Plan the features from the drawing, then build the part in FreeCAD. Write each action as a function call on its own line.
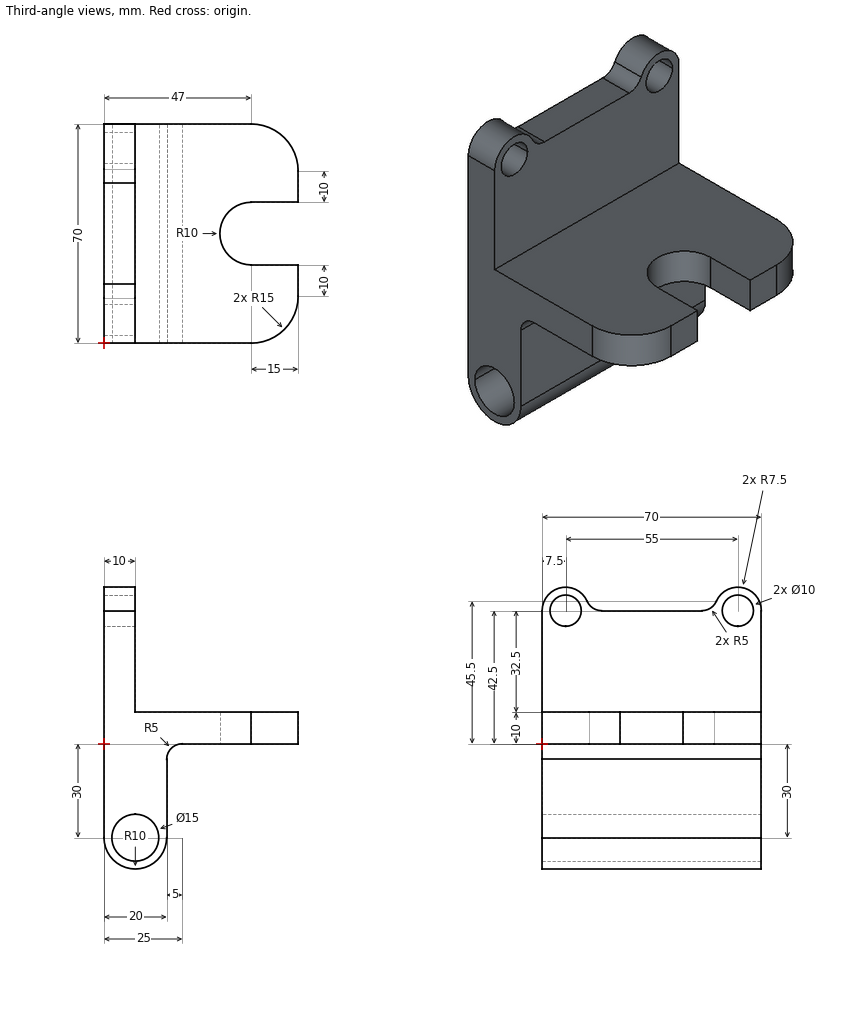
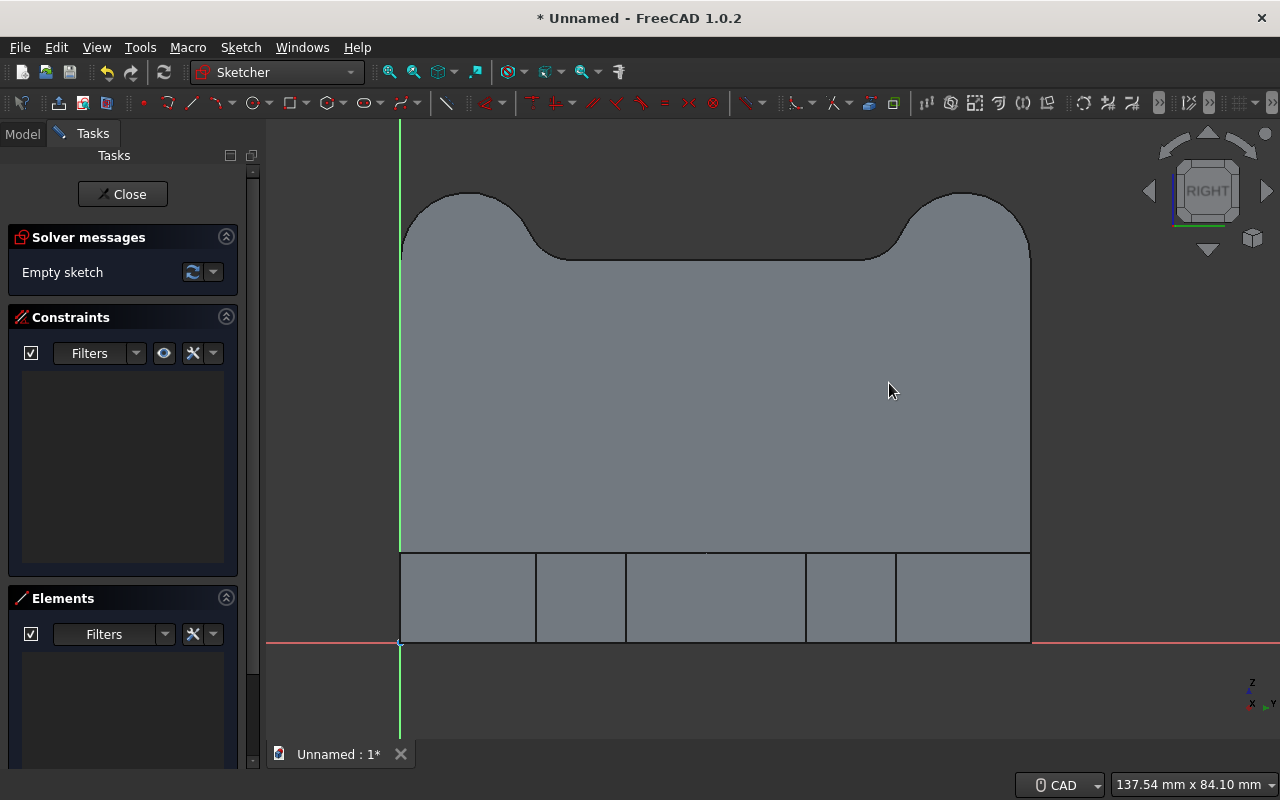
click(254, 104)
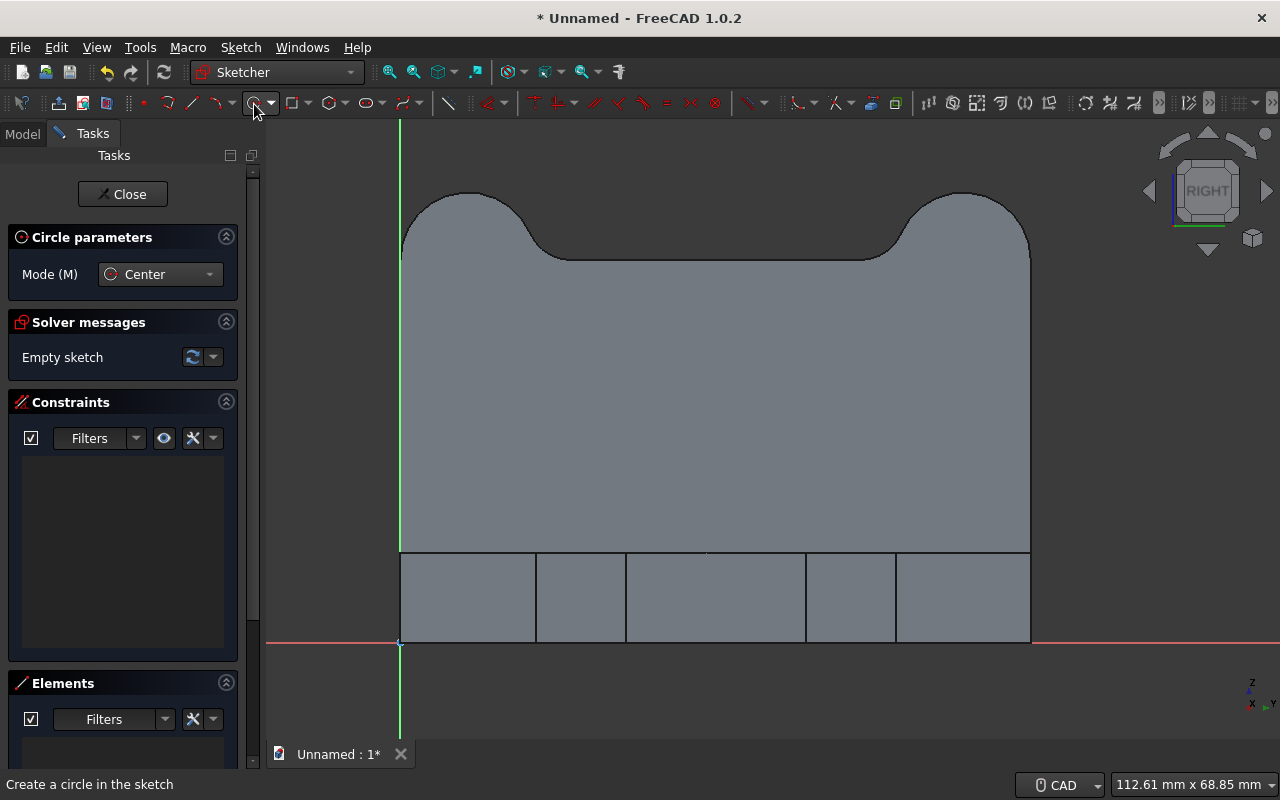
click(963, 260)
click(995, 228)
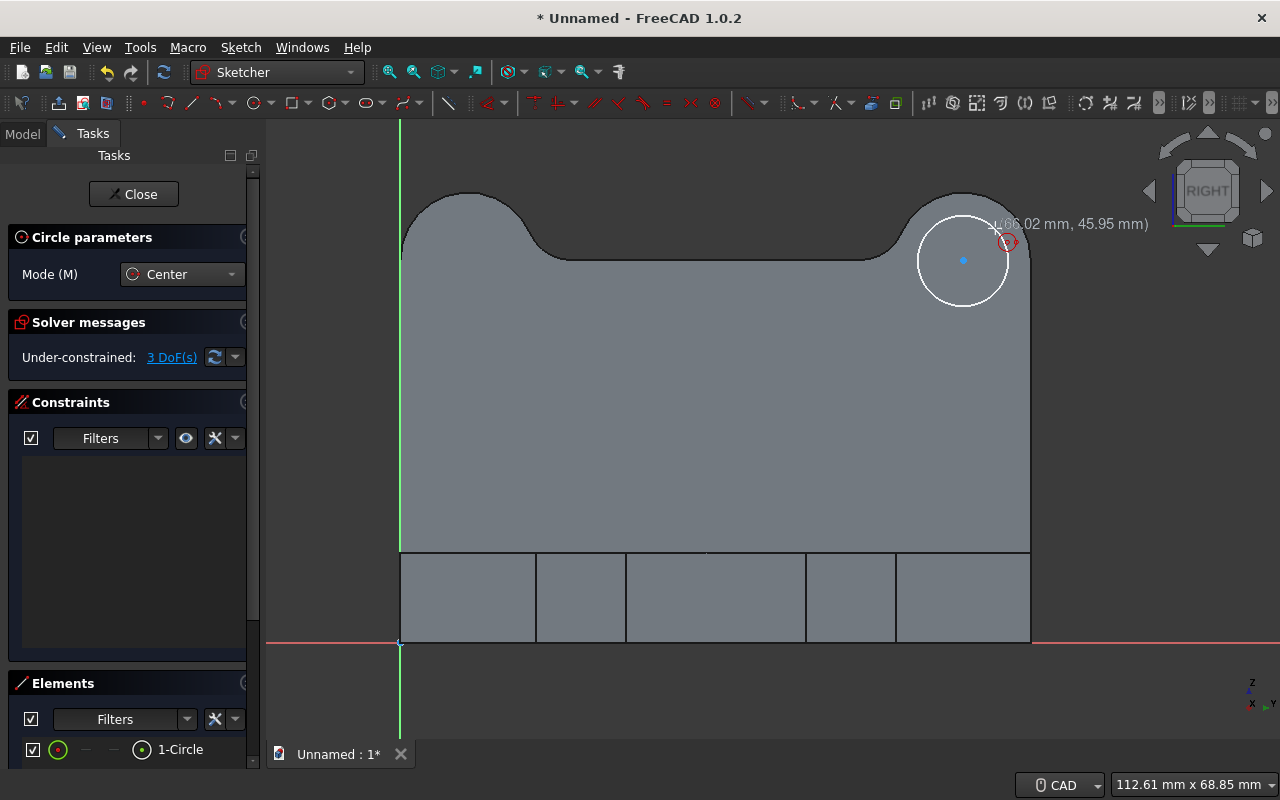
click(468, 260)
click(500, 228)
key(Escape)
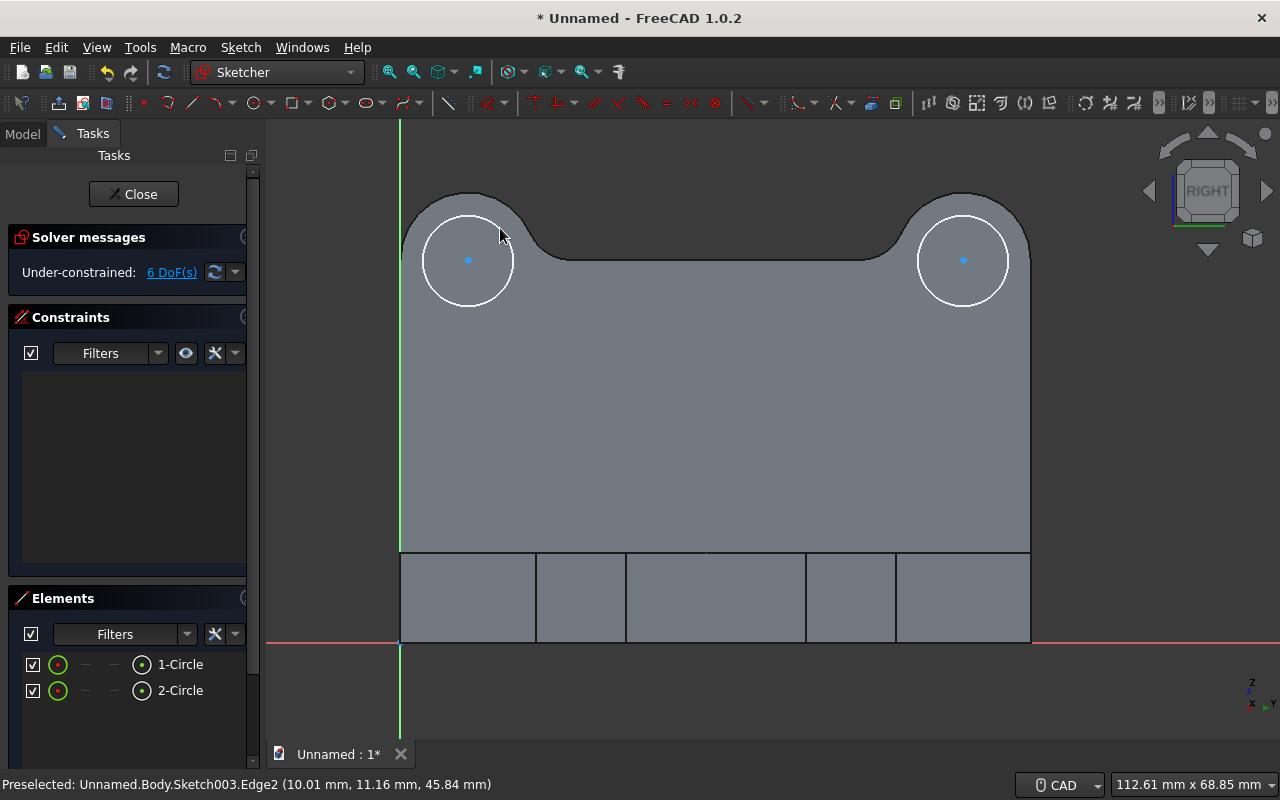
click(995, 229)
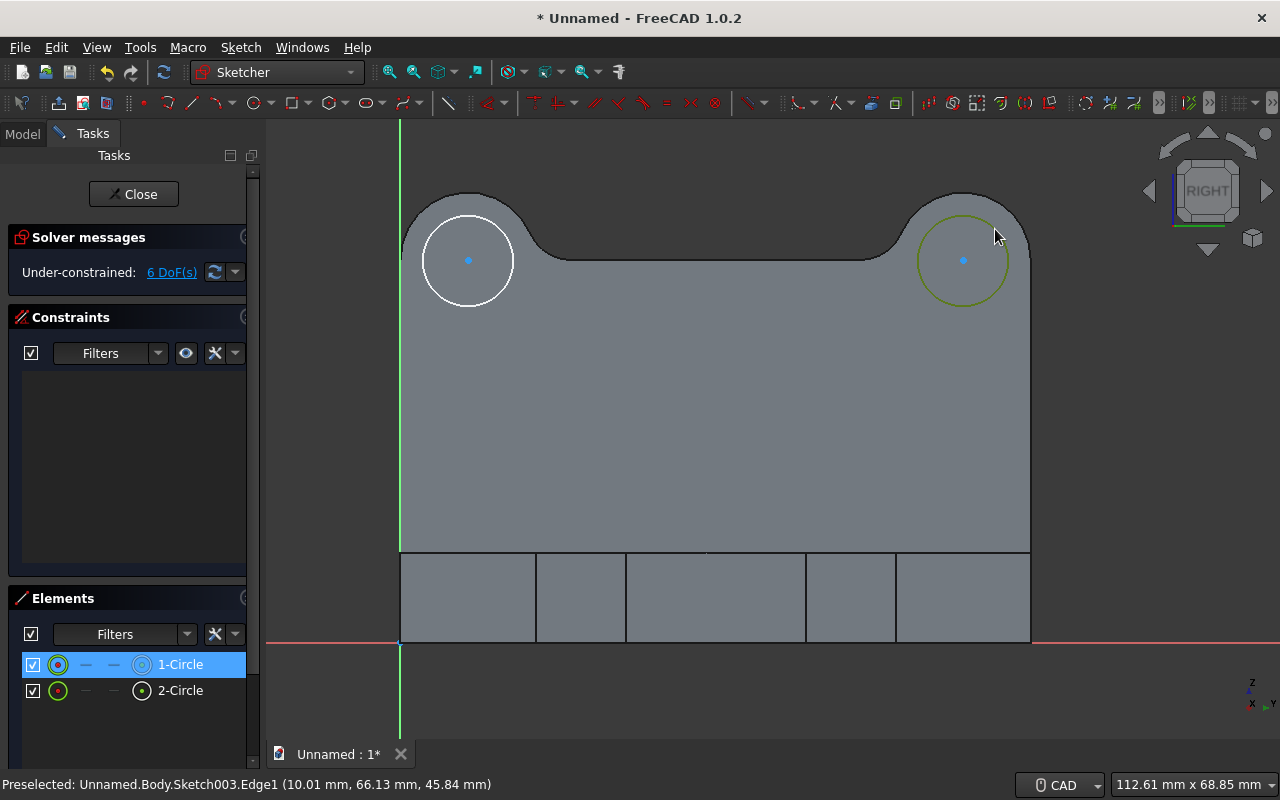
click(500, 229)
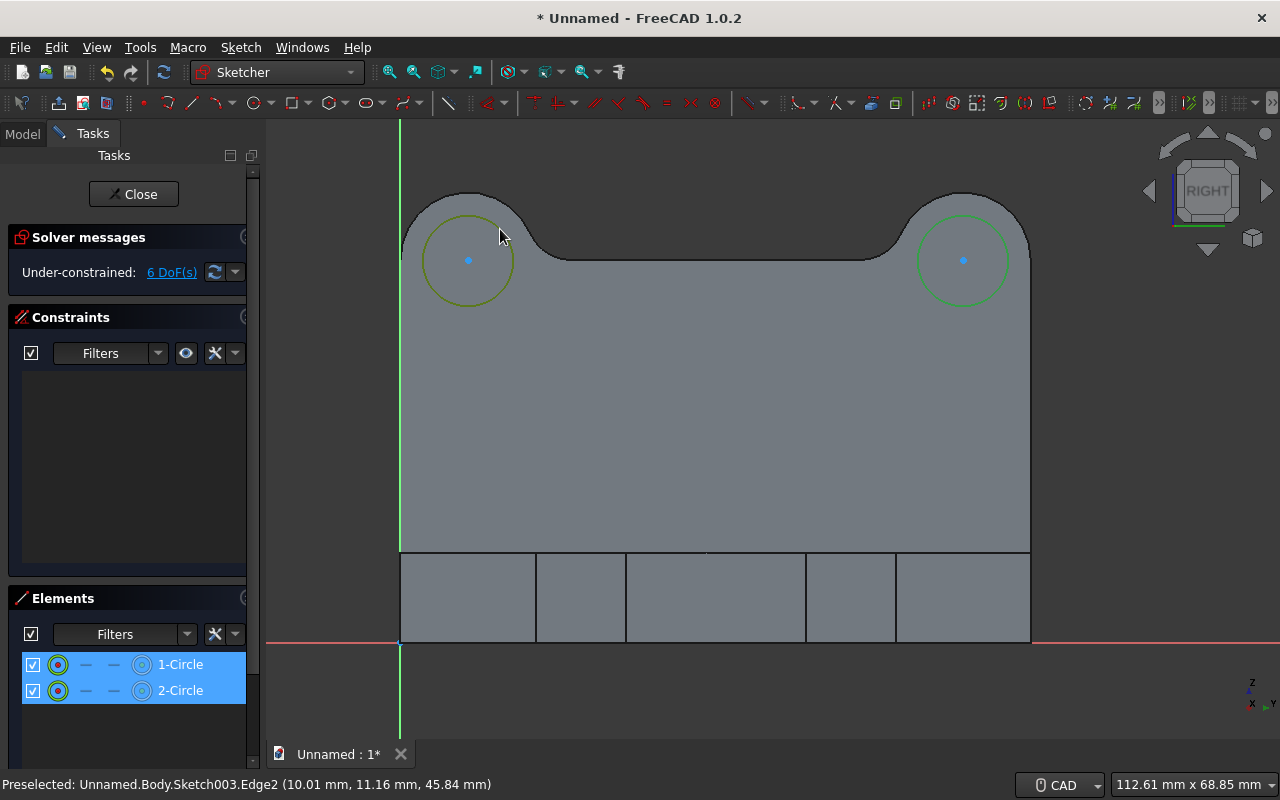
click(668, 104)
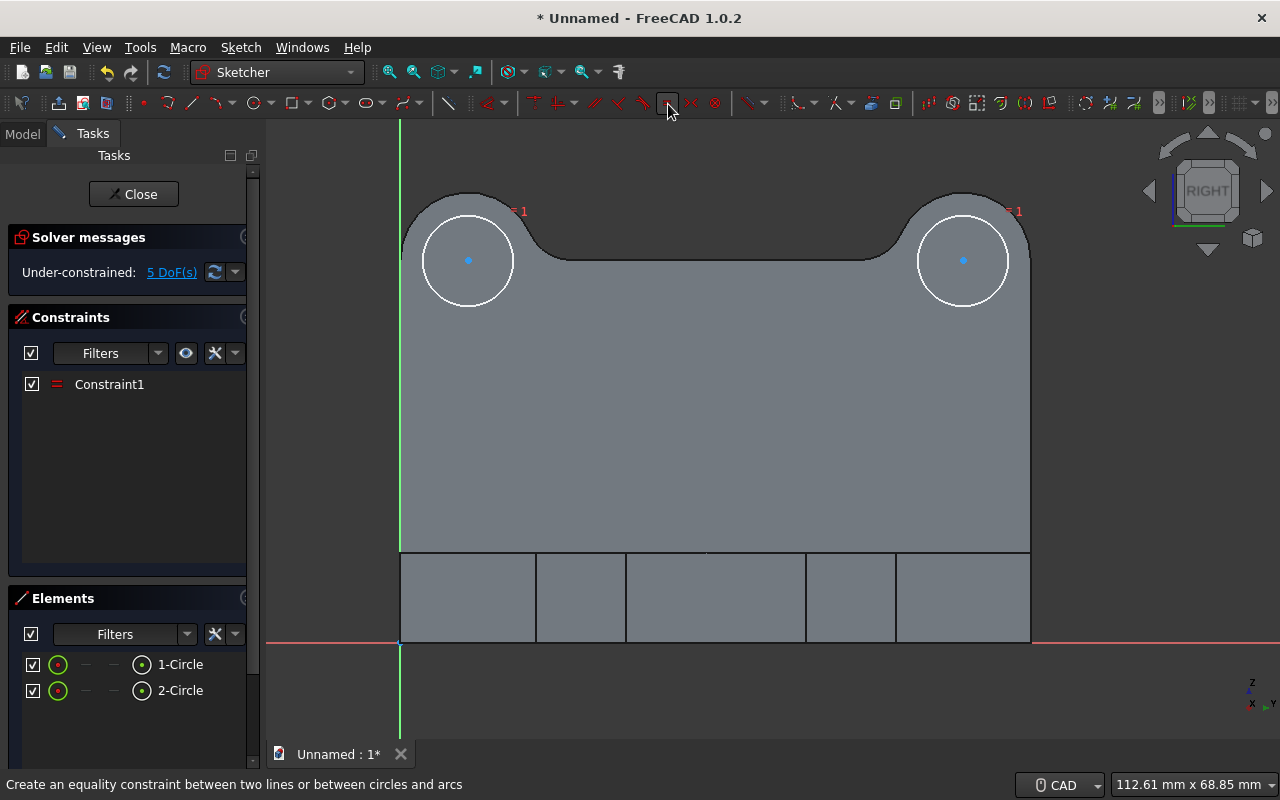
click(963, 261)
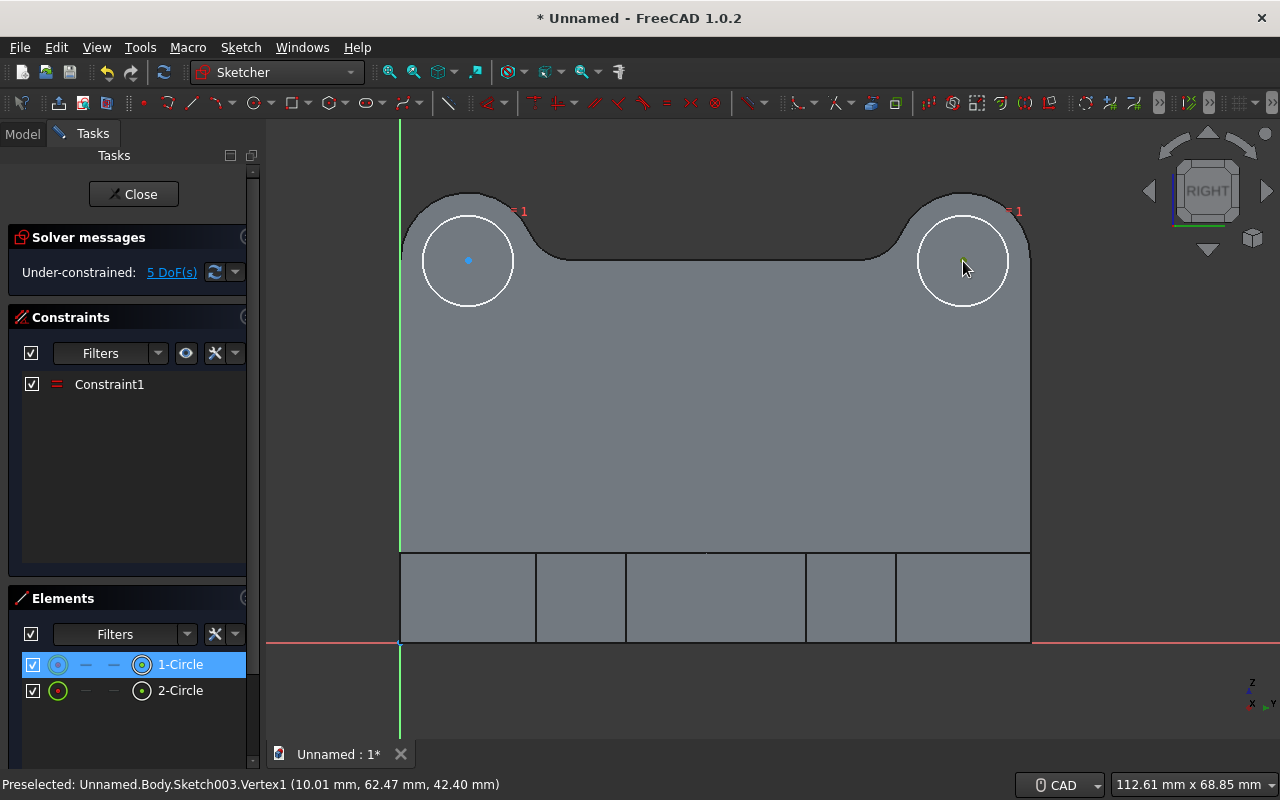
click(468, 261)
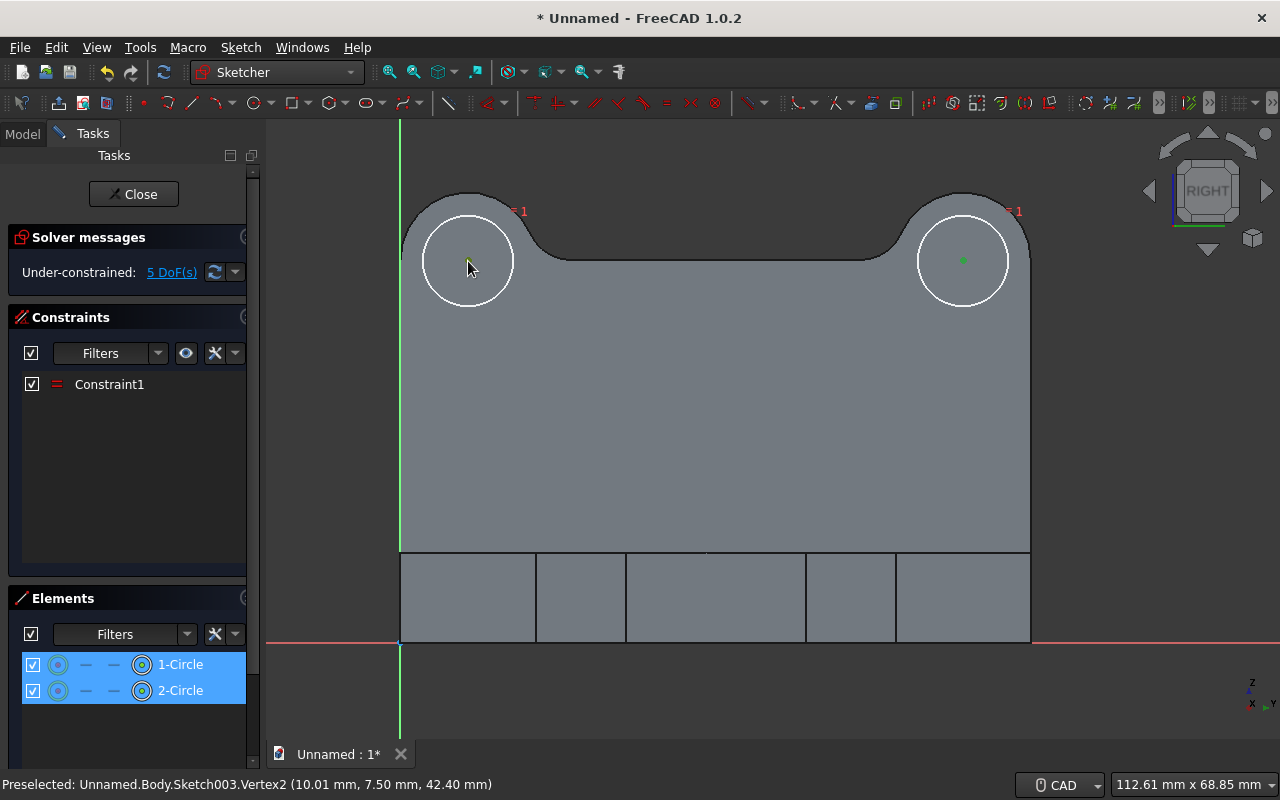
key(h)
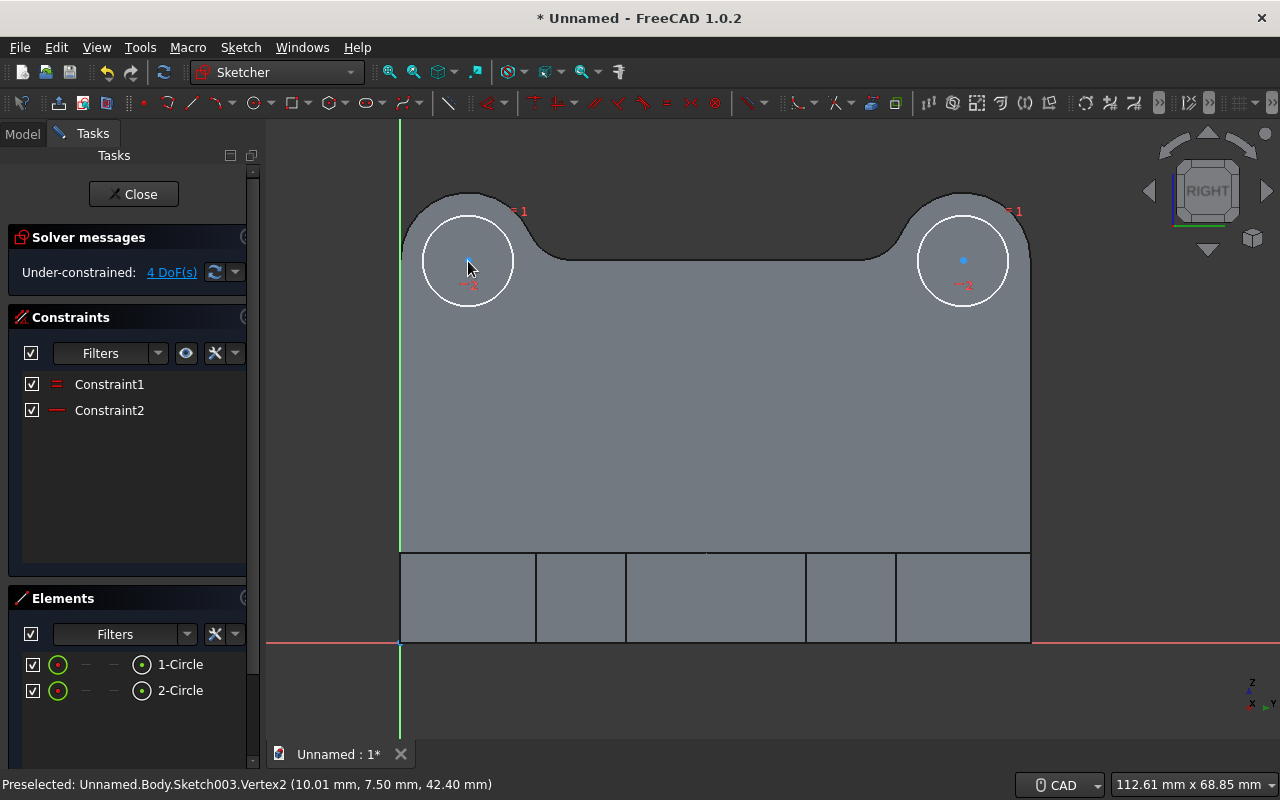
click(488, 104)